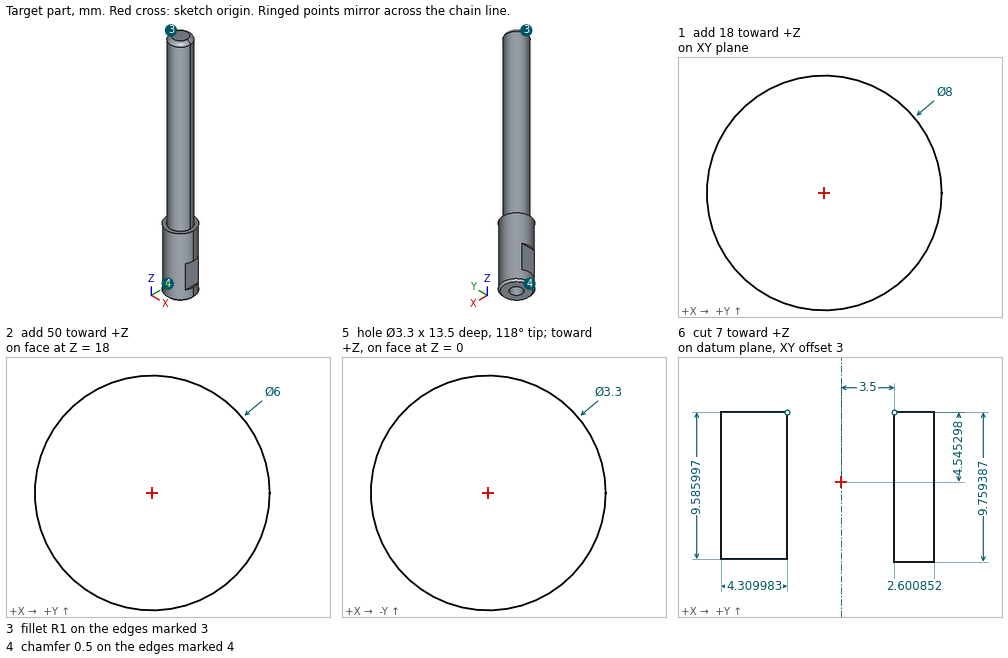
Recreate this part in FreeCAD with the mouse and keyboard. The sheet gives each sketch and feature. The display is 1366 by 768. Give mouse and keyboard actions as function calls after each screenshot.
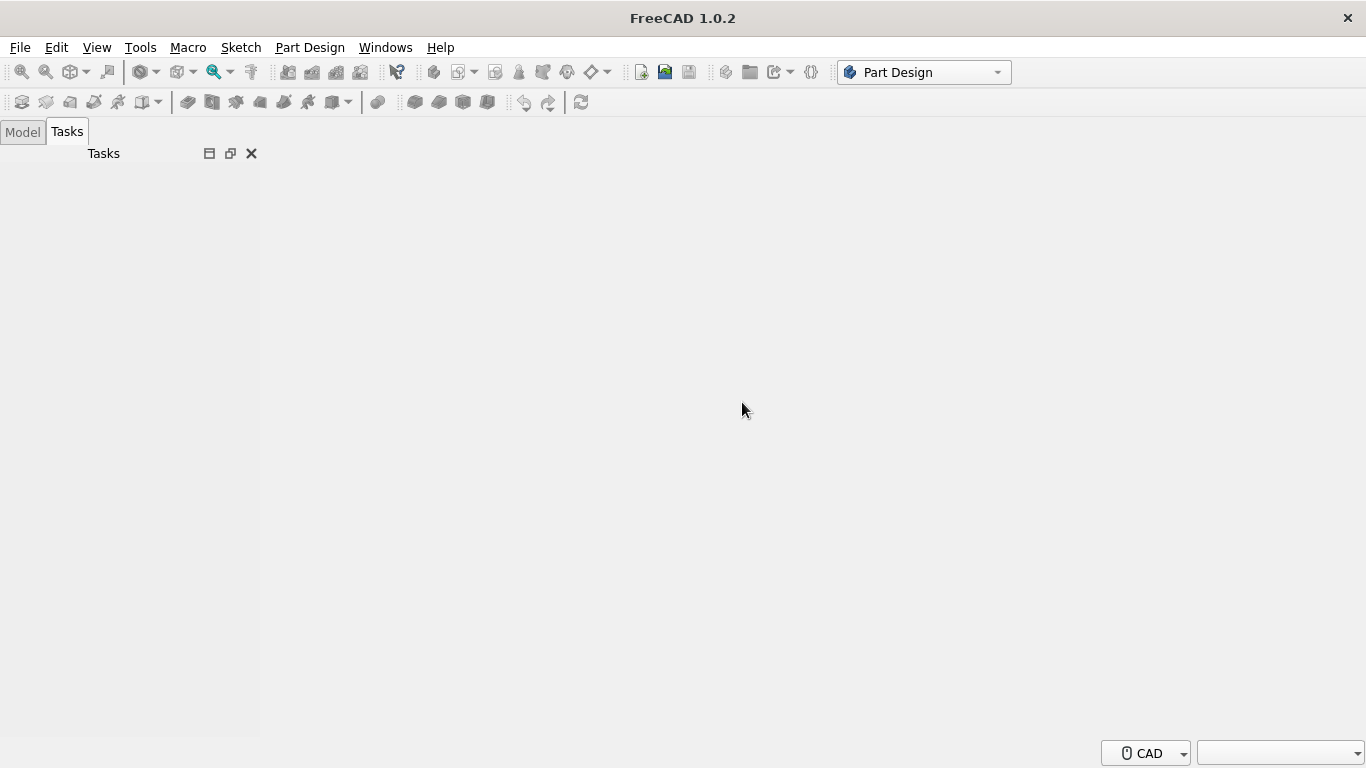
click(642, 72)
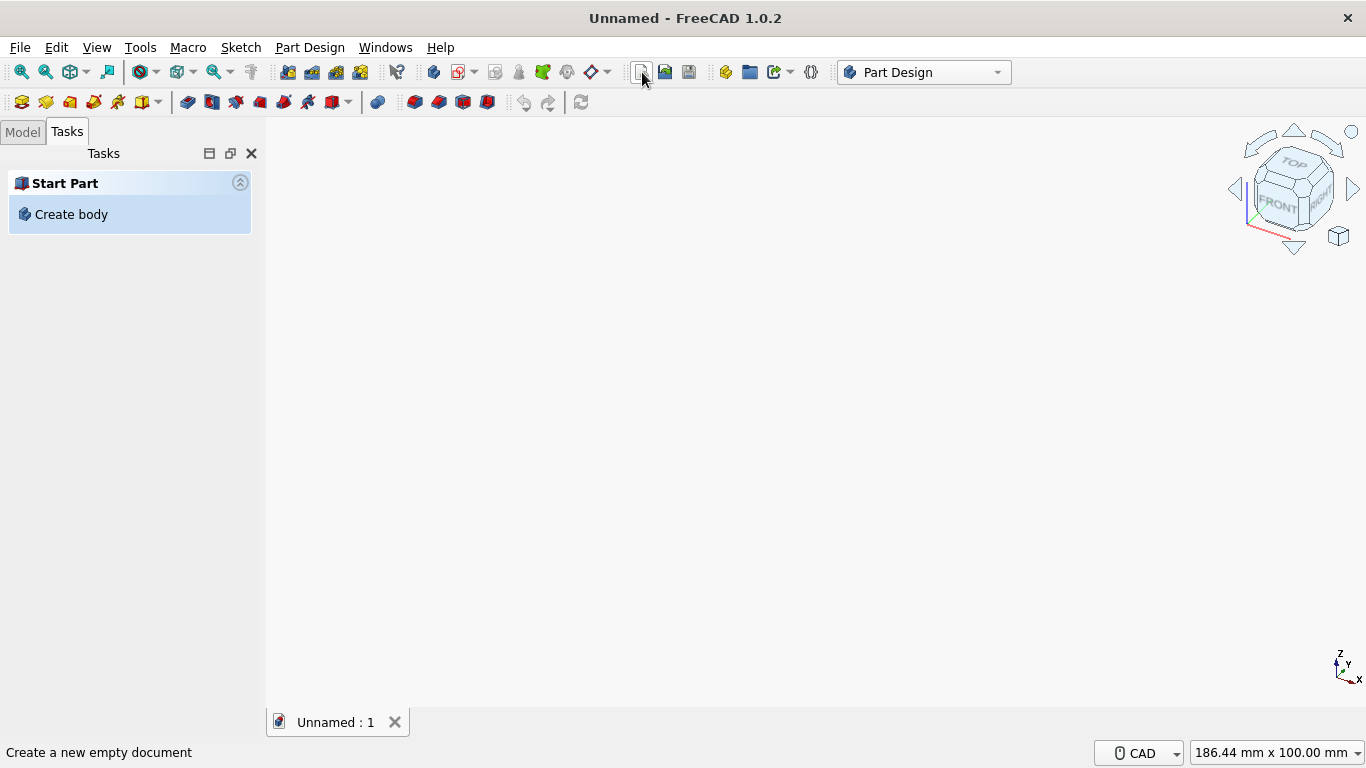
click(458, 72)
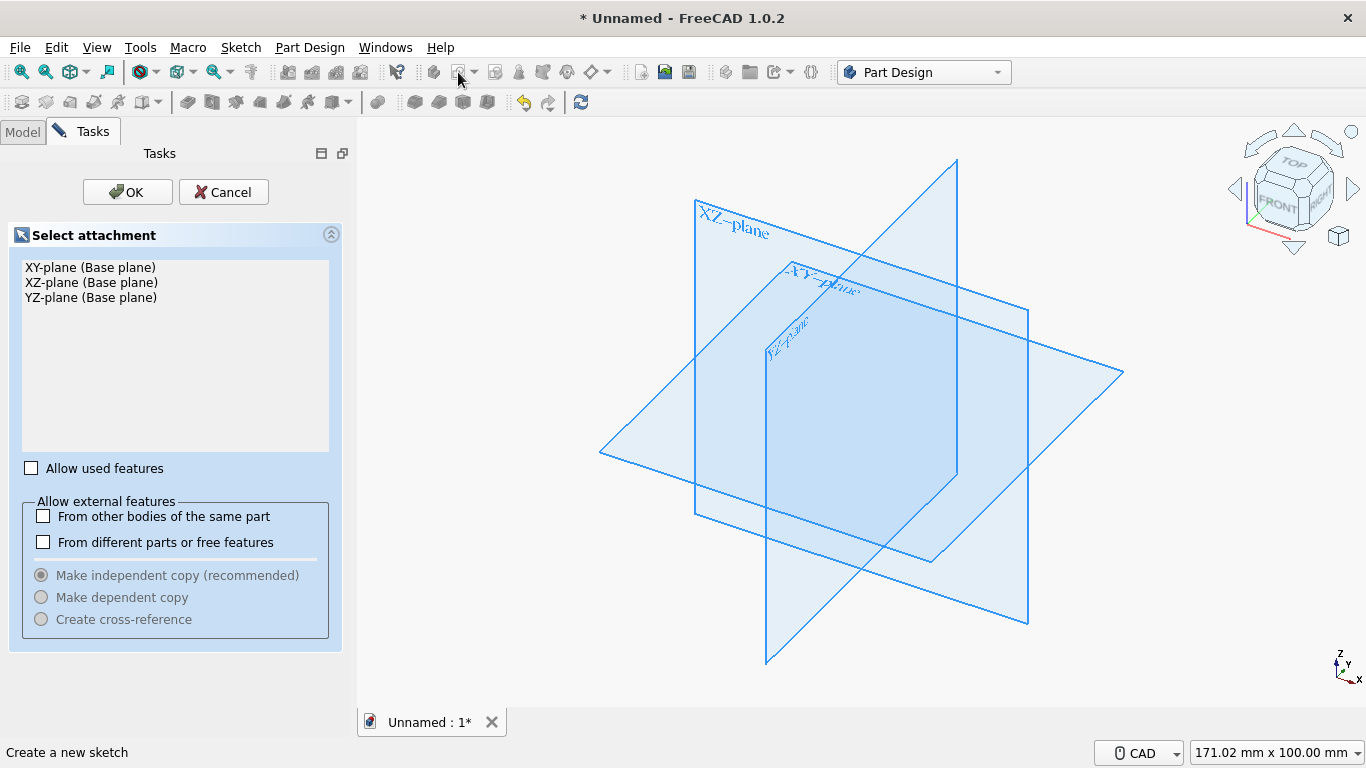
click(82, 268)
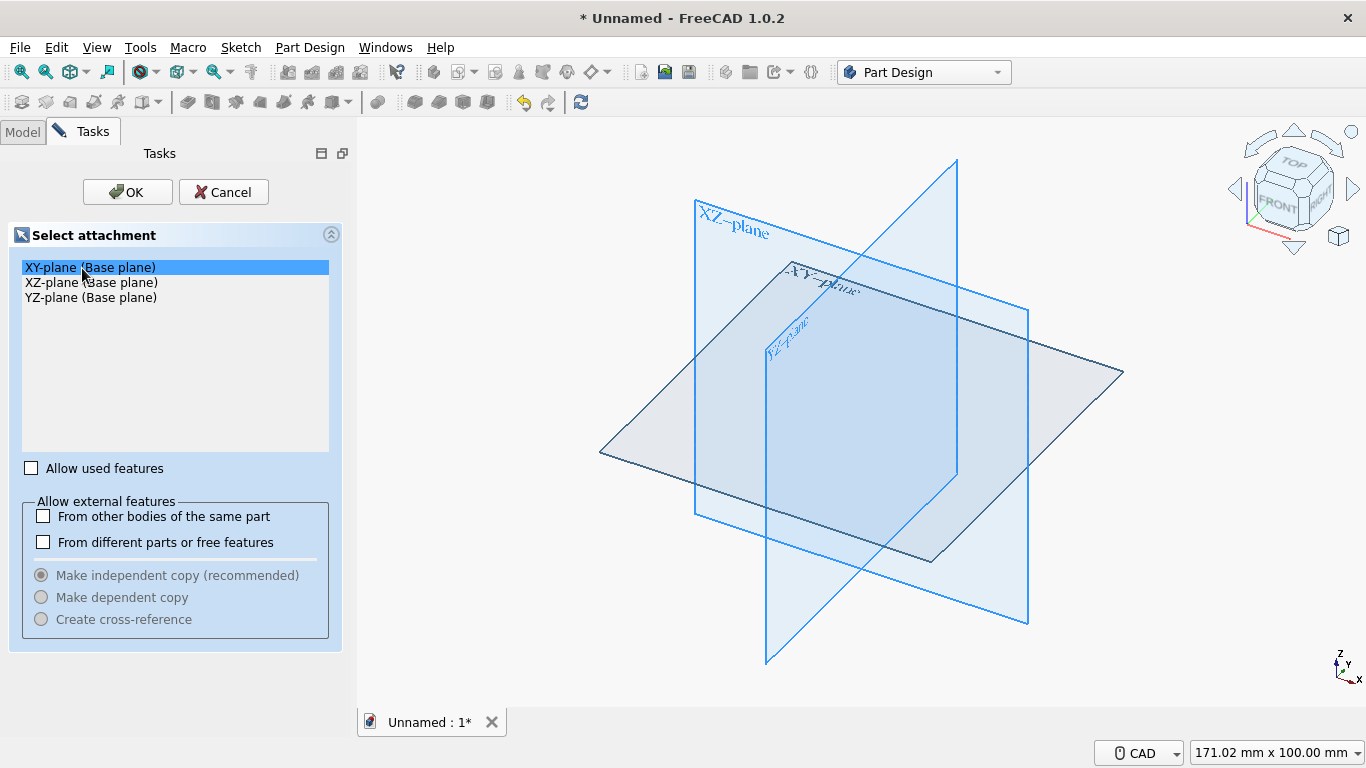
click(128, 192)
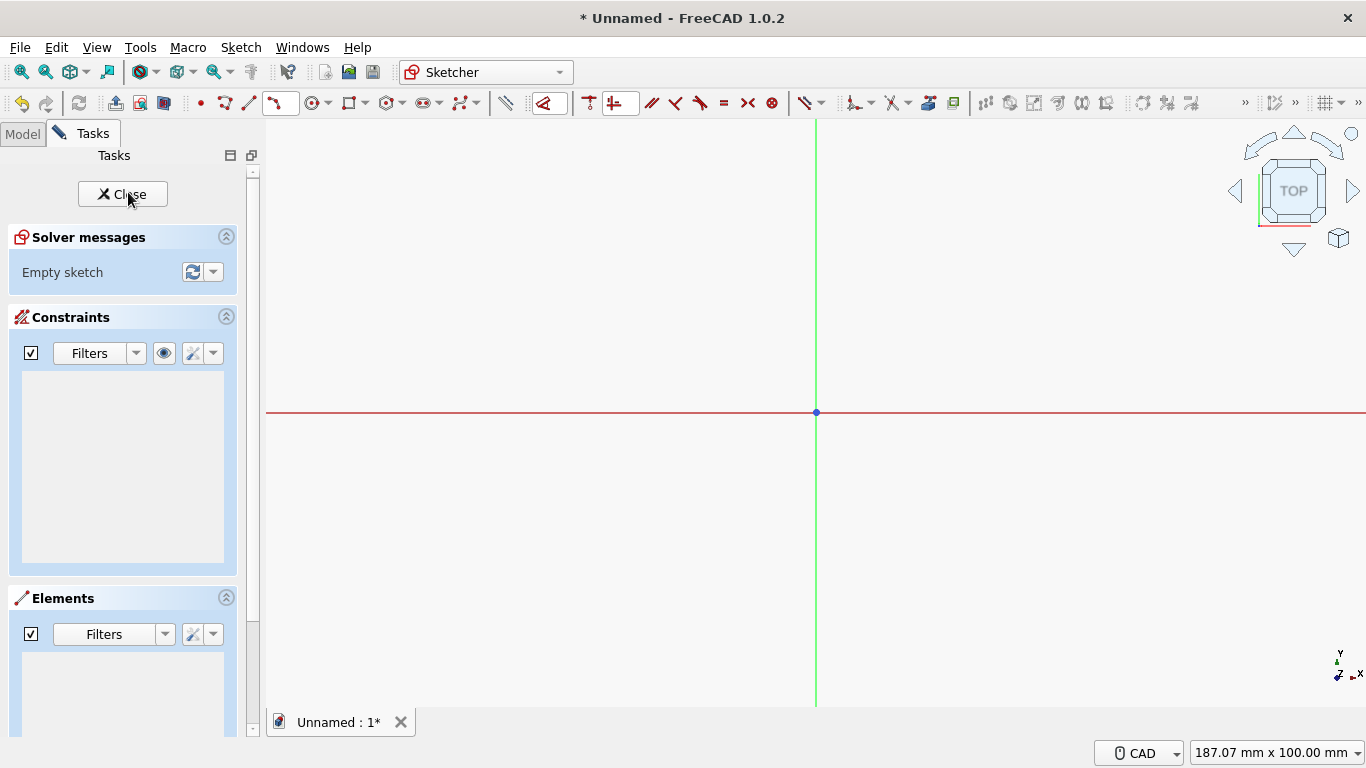
scroll(827, 413, up, 10)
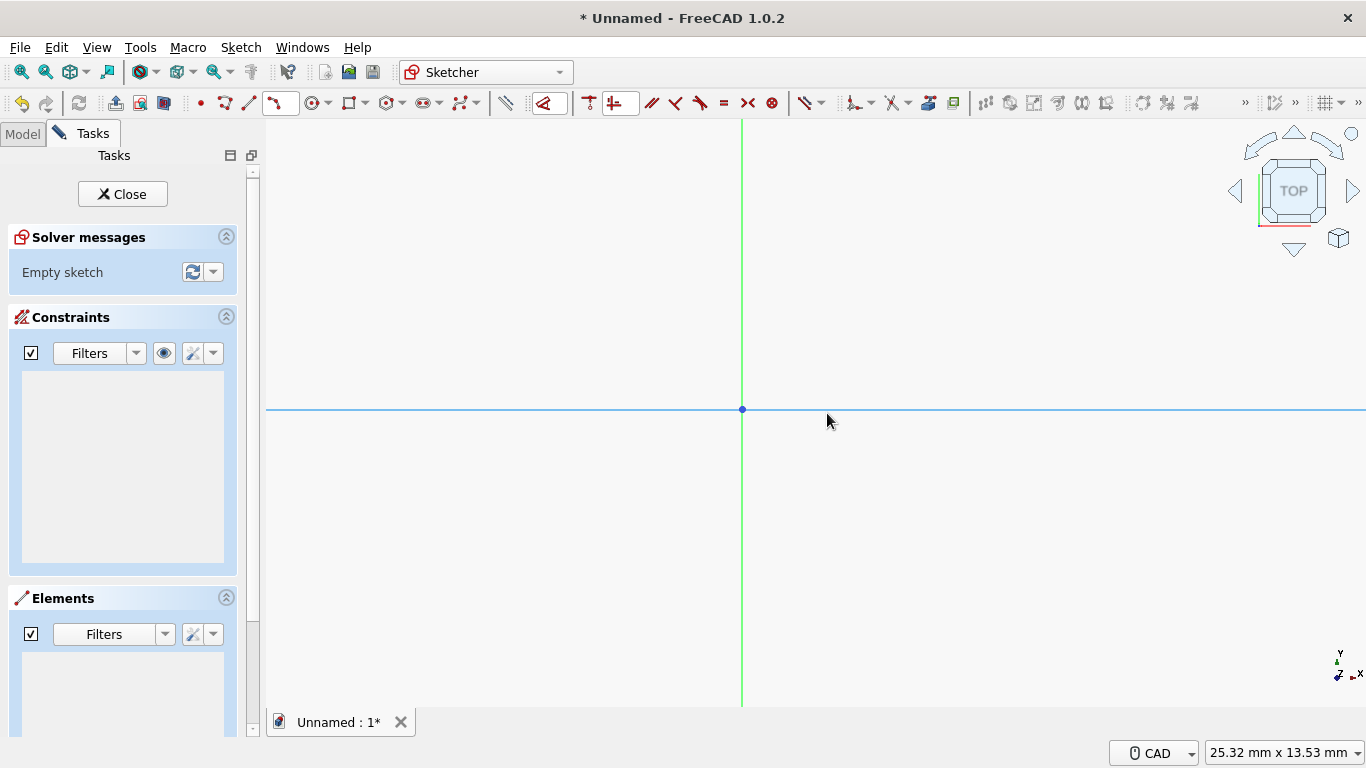
click(312, 104)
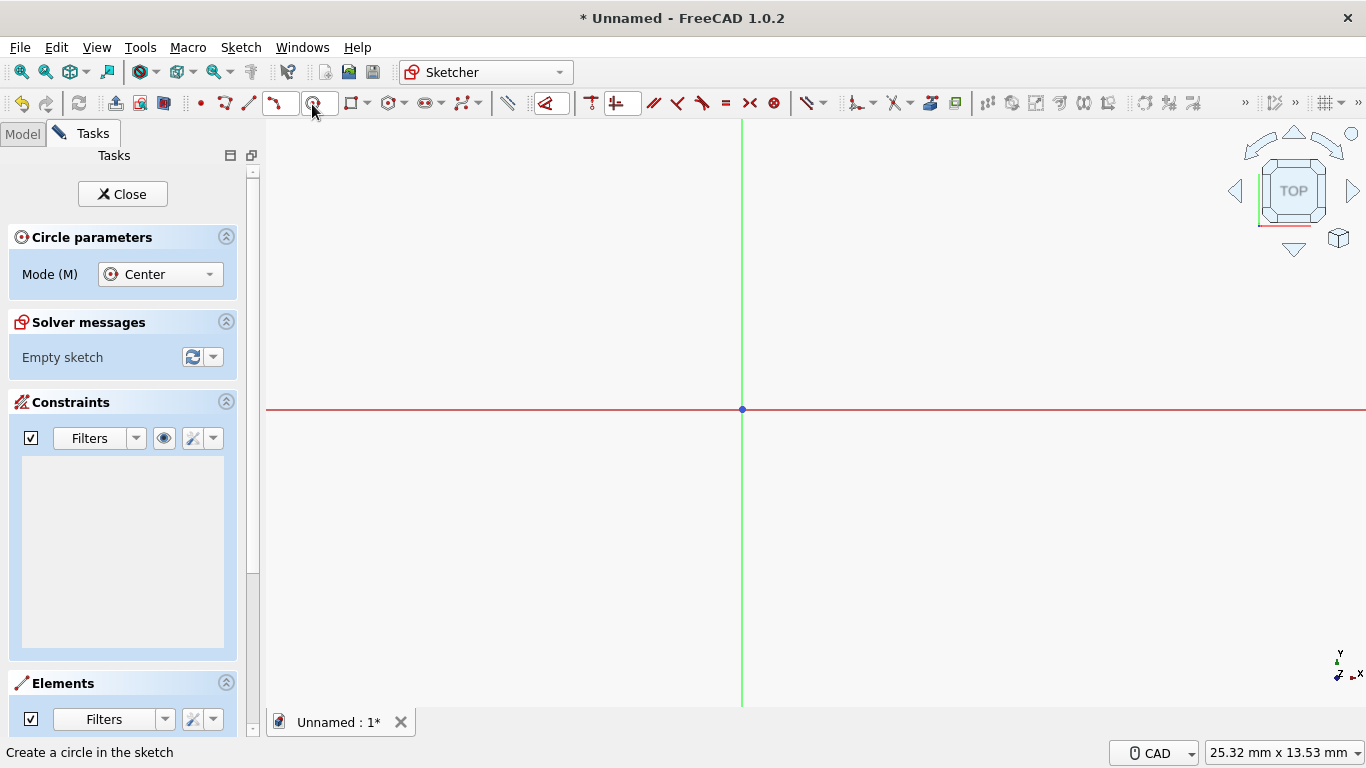
click(742, 410)
move(865, 287)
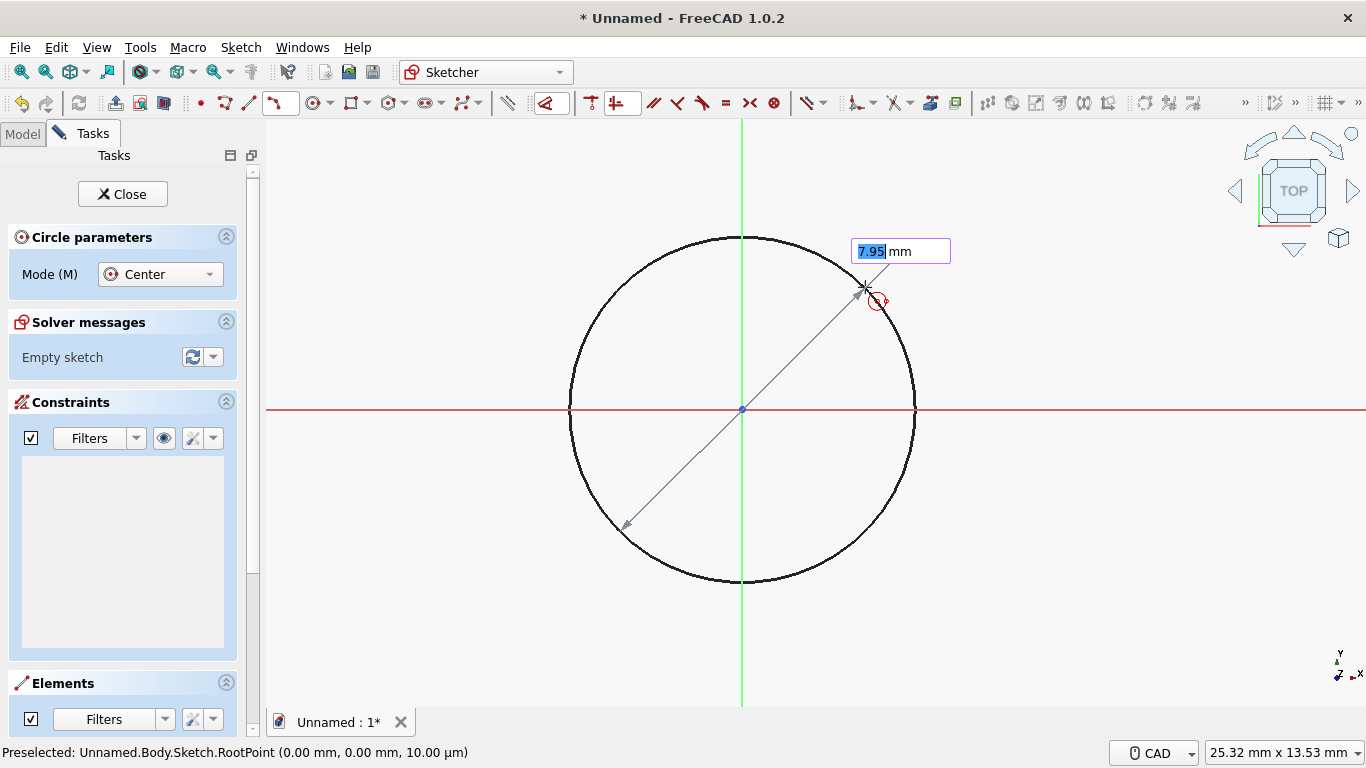
text(8)
key(Return)
key(Escape)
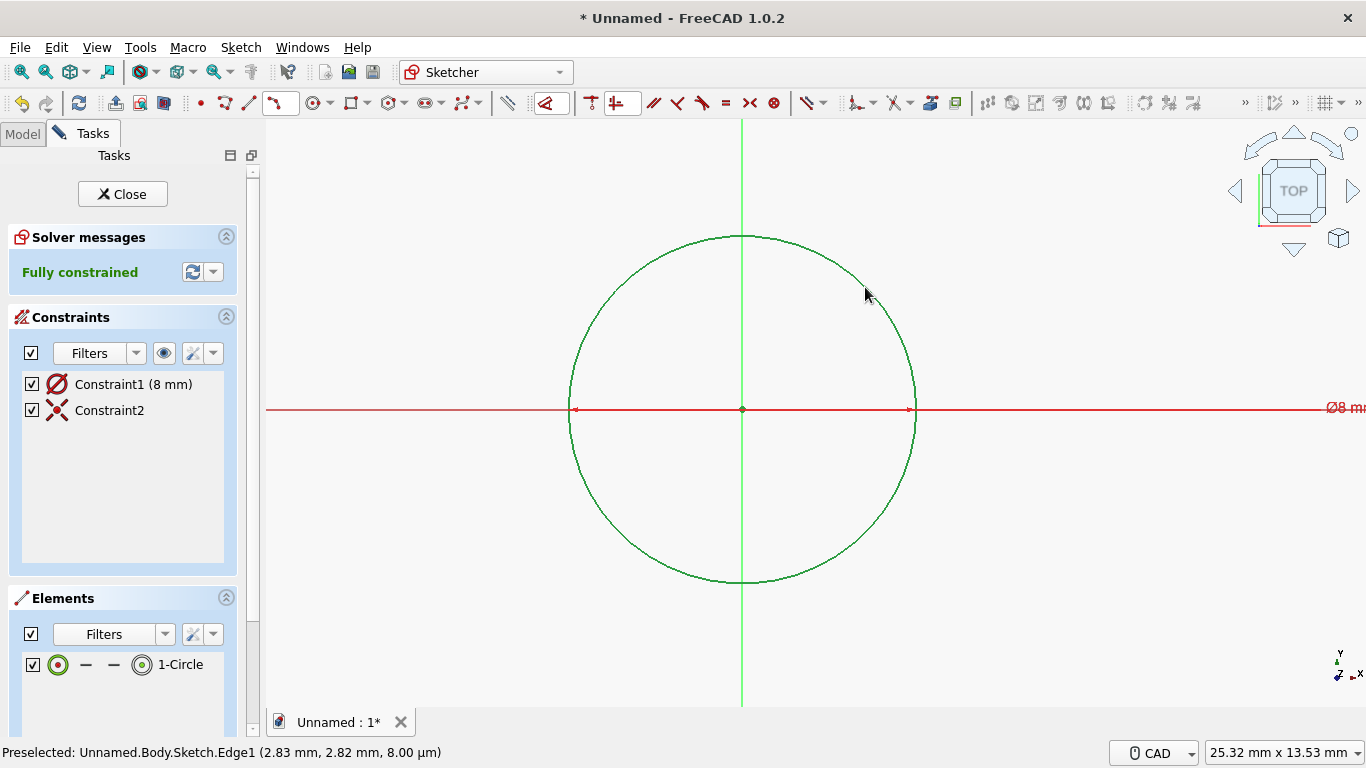
click(123, 194)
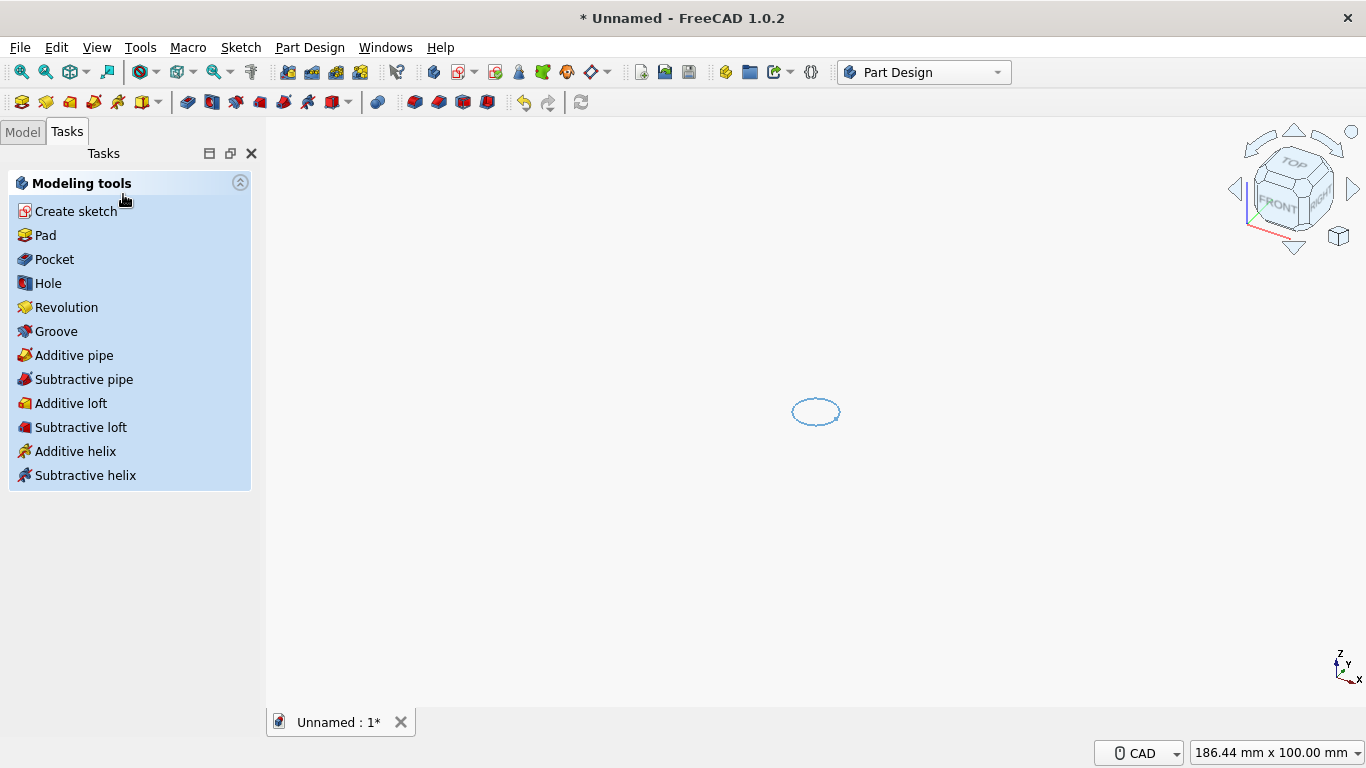
click(22, 102)